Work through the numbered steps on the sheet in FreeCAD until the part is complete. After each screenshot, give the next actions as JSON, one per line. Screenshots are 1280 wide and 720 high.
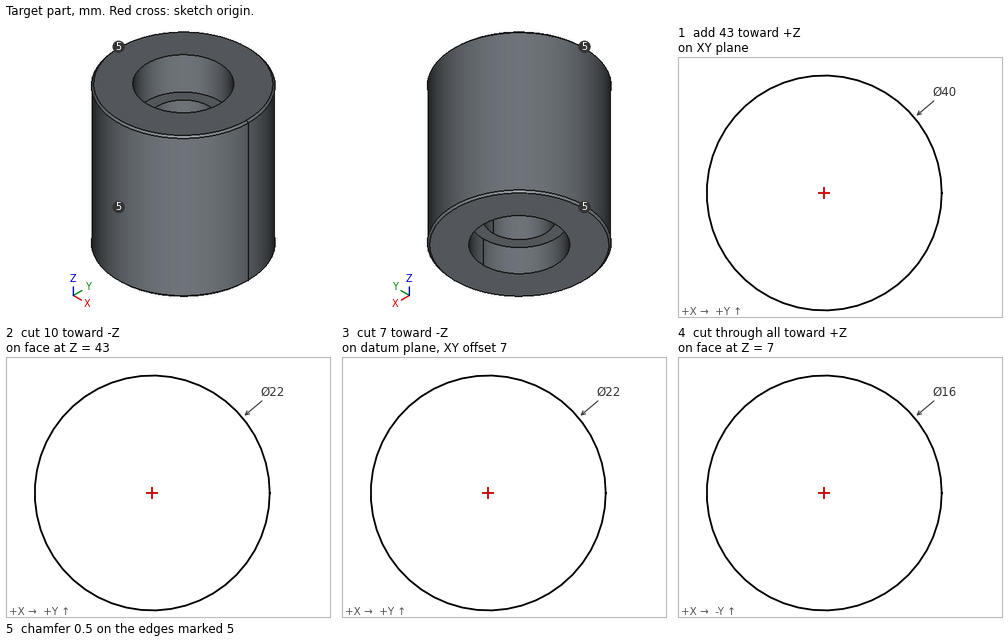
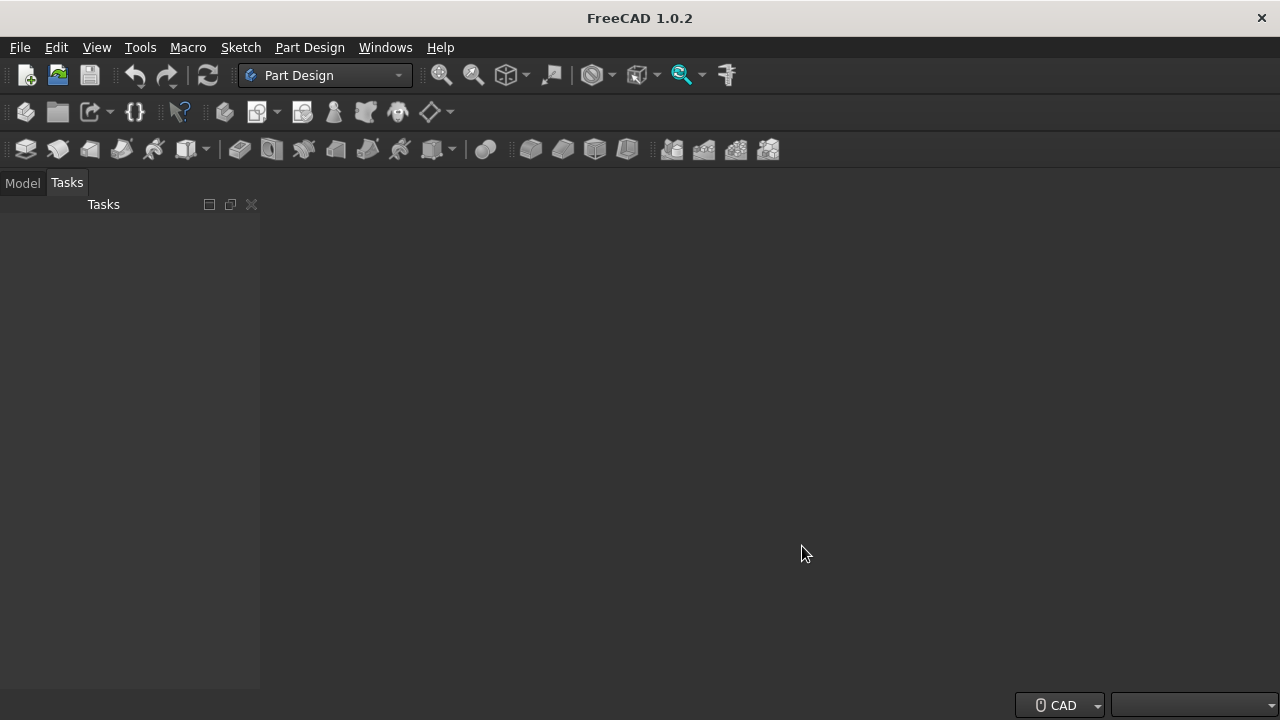
{"action": "left_click", "coordinate": [26, 76]}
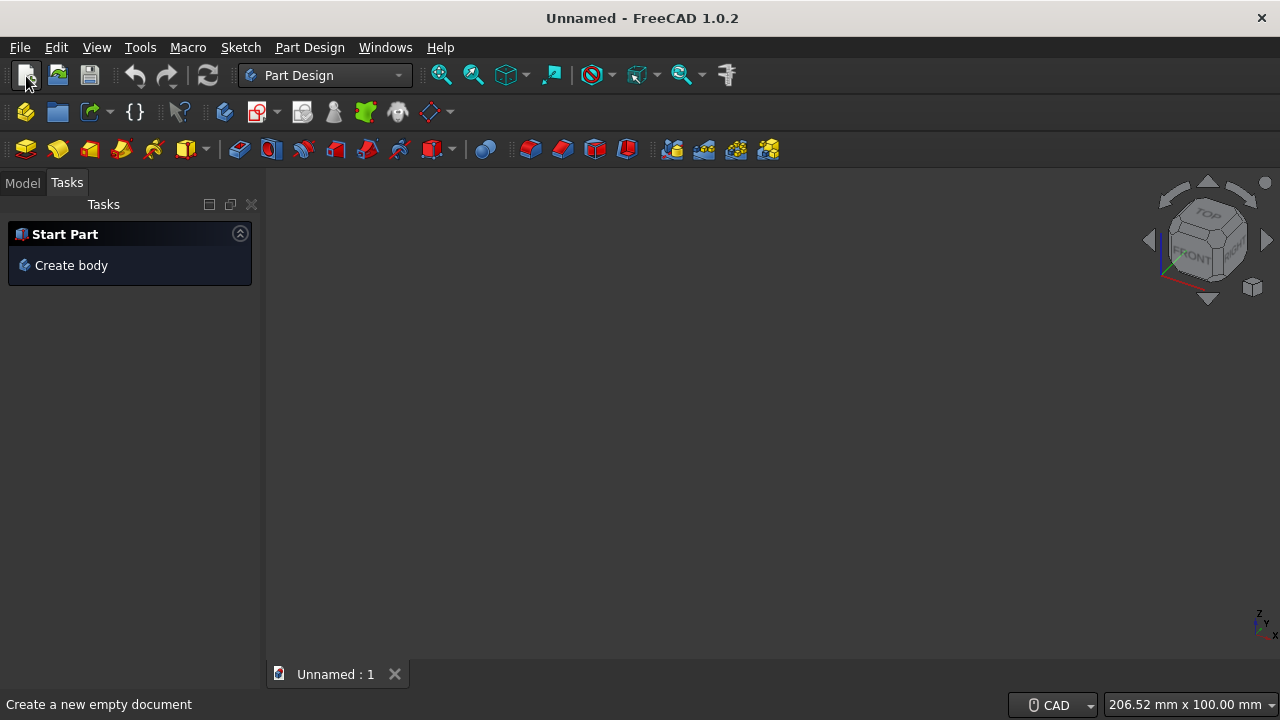
{"action": "left_click", "coordinate": [258, 112]}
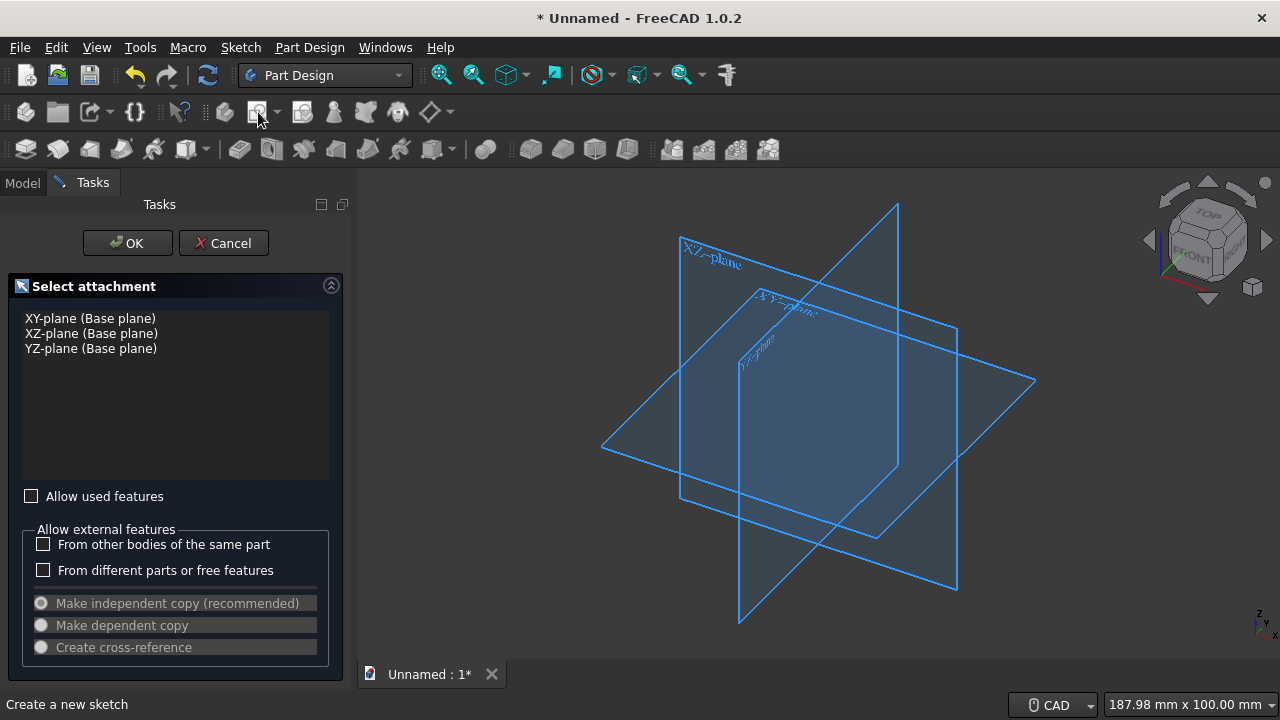
{"action": "left_click", "coordinate": [82, 318]}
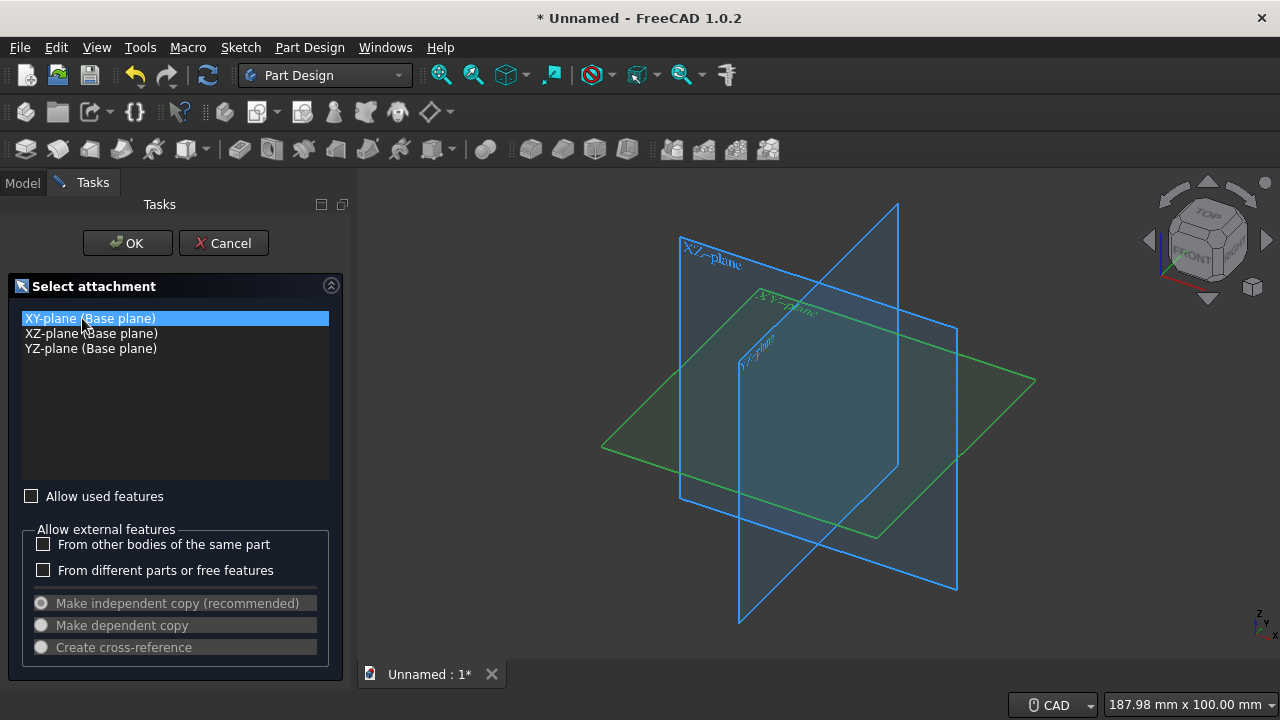
{"action": "left_click", "coordinate": [128, 243]}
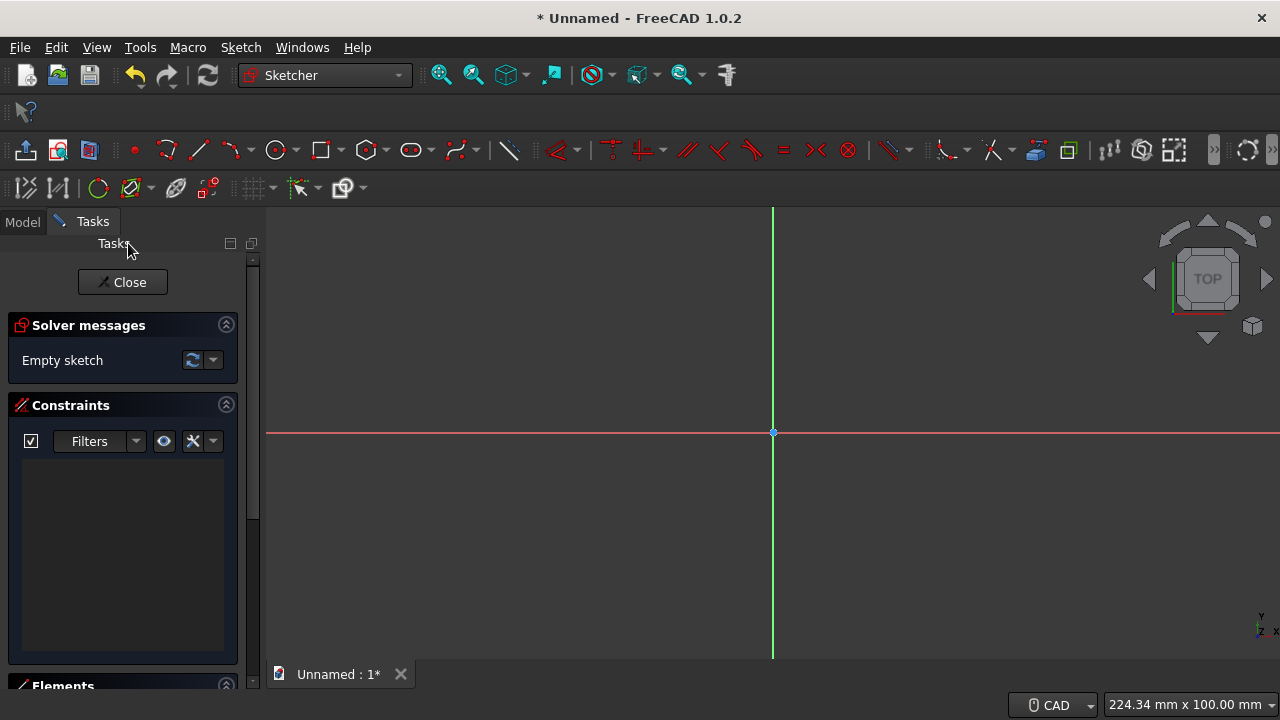
{"action": "scroll", "coordinate": [912, 433], "scroll_direction": "up", "scroll_amount": 2}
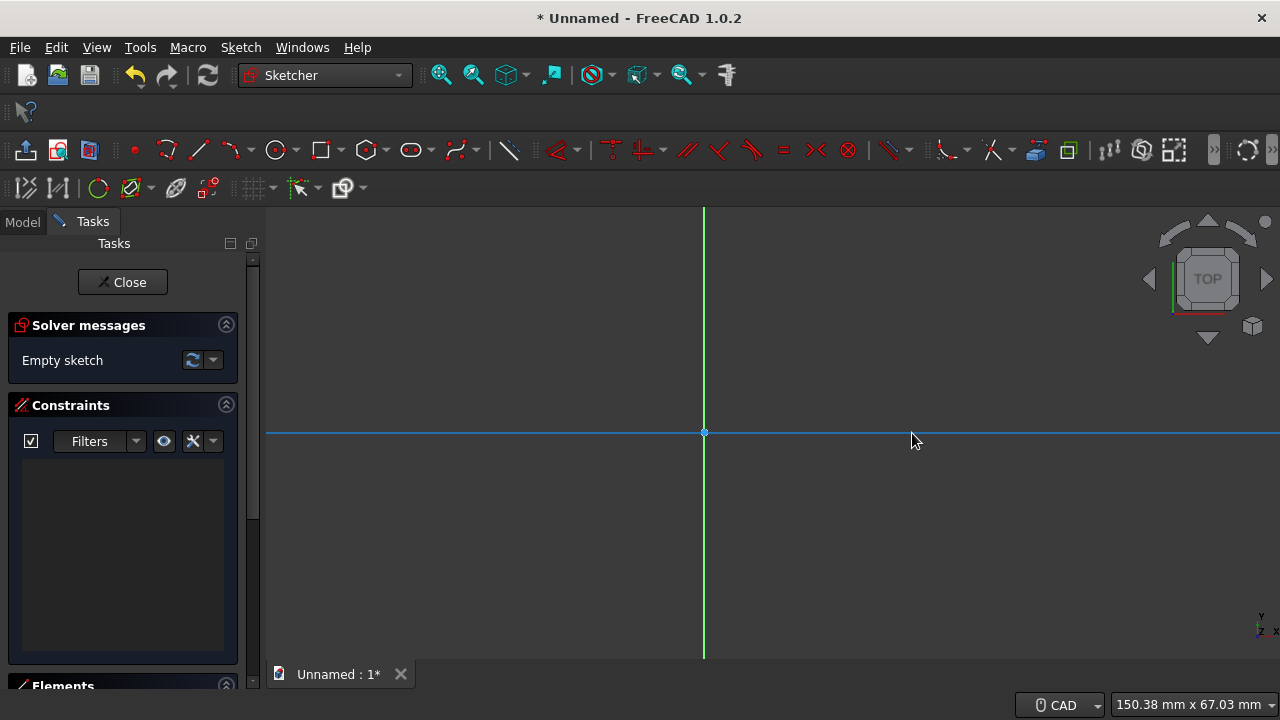
{"action": "left_click", "coordinate": [276, 150]}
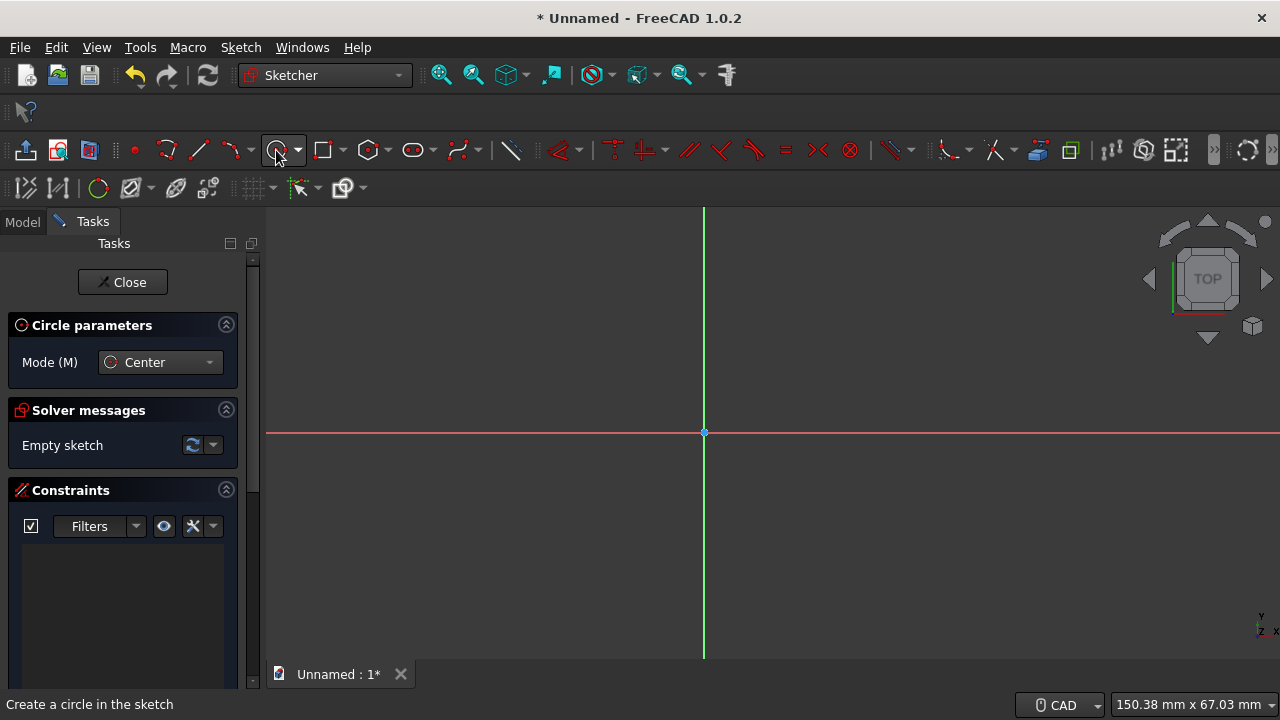
{"action": "left_click", "coordinate": [704, 433]}
{"action": "mouse_move", "coordinate": [800, 337]}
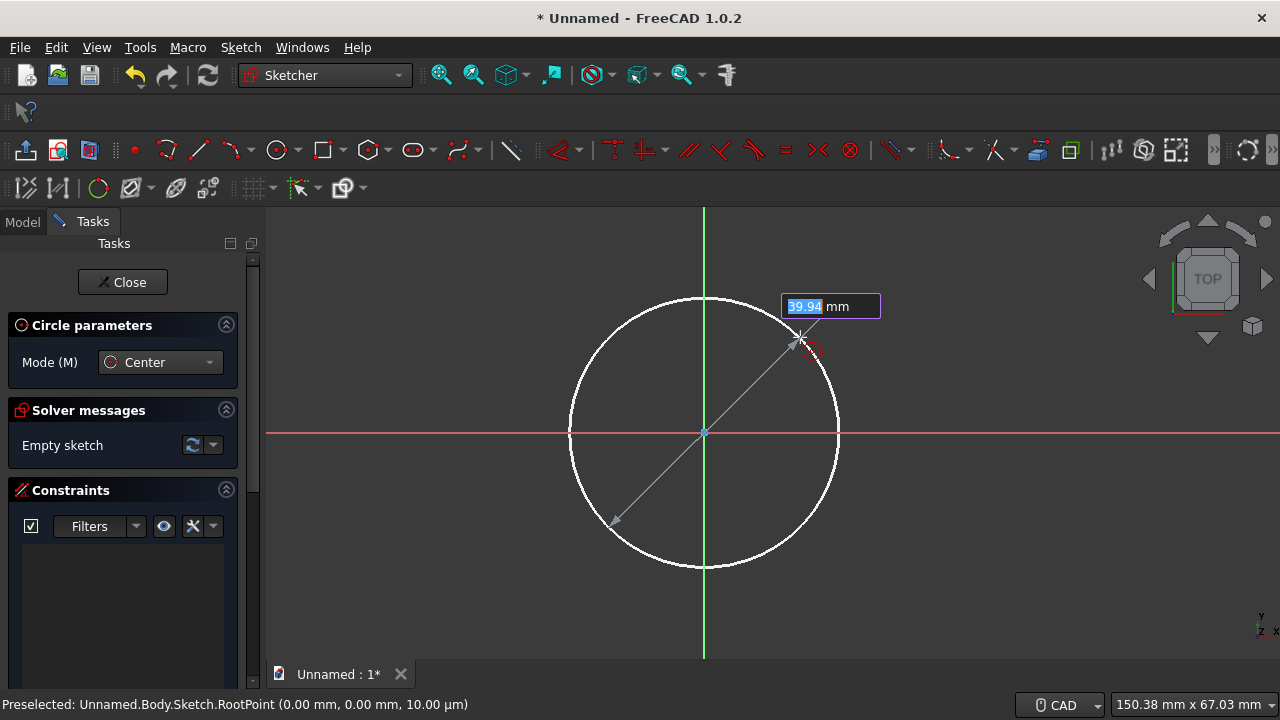
{"action": "type", "text": "40"}
{"action": "key", "text": "Return"}
{"action": "key", "text": "Escape"}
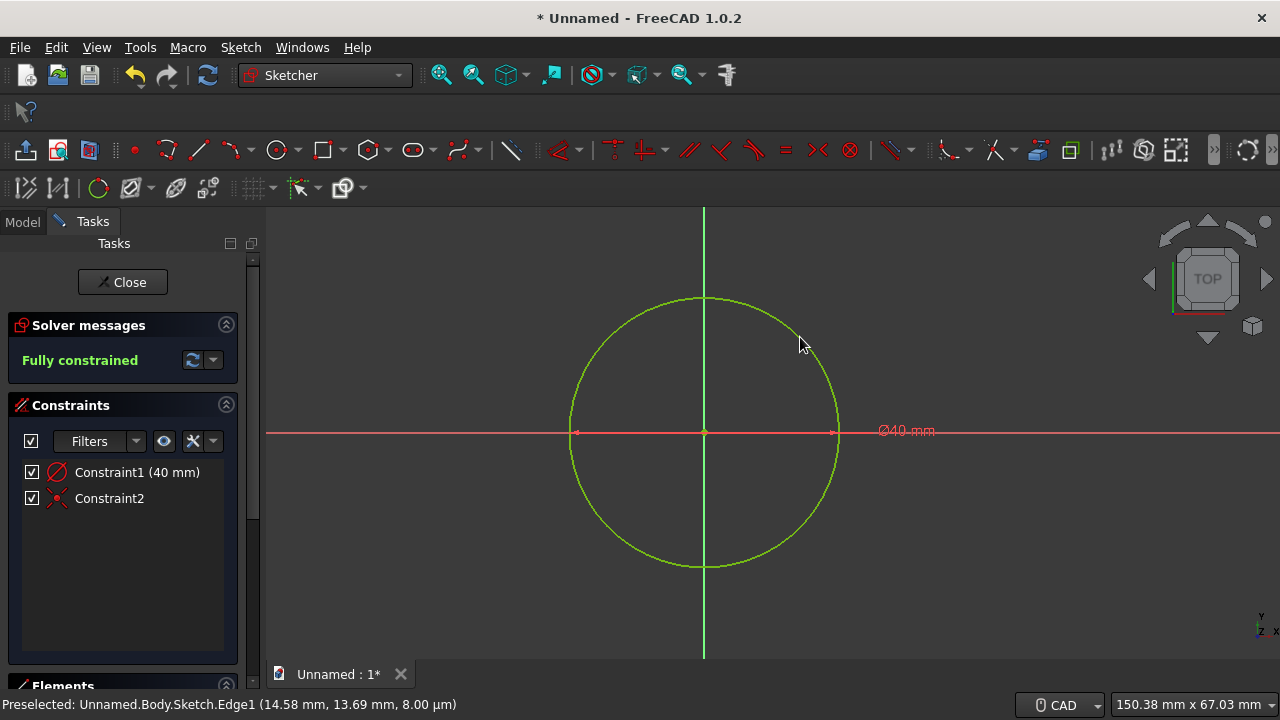
{"action": "left_click", "coordinate": [123, 282]}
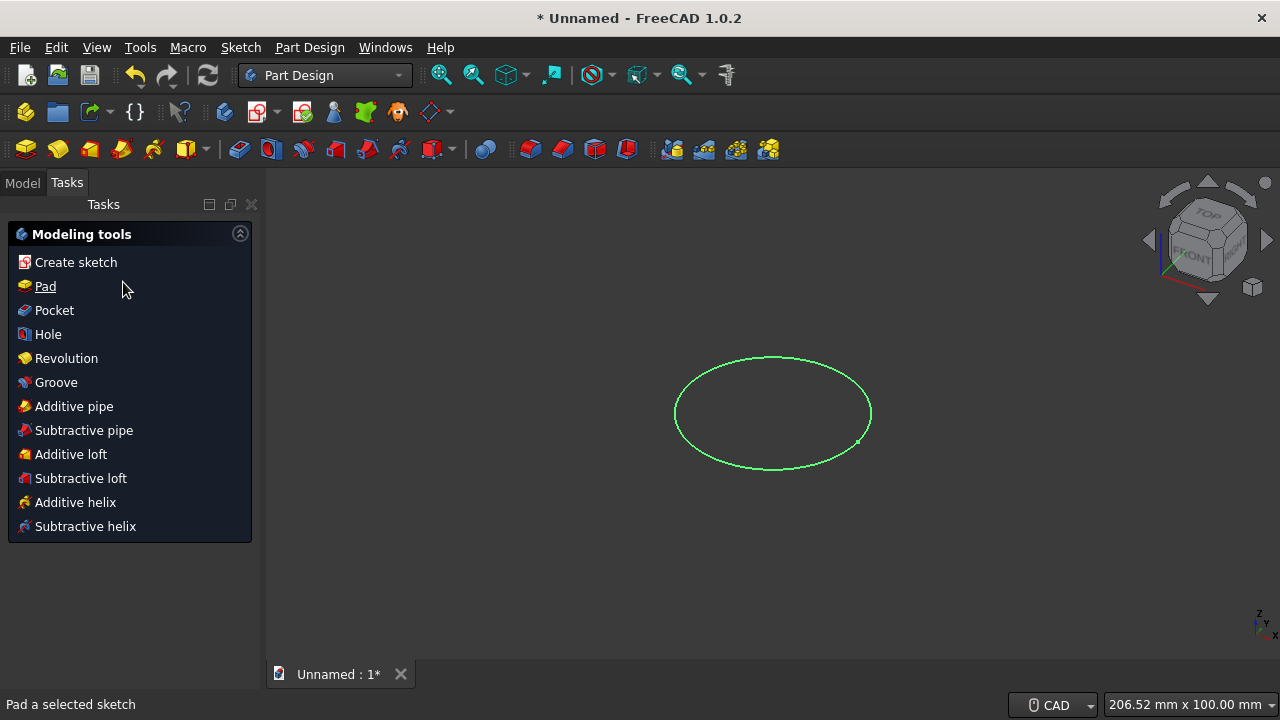
{"action": "left_click", "coordinate": [26, 150]}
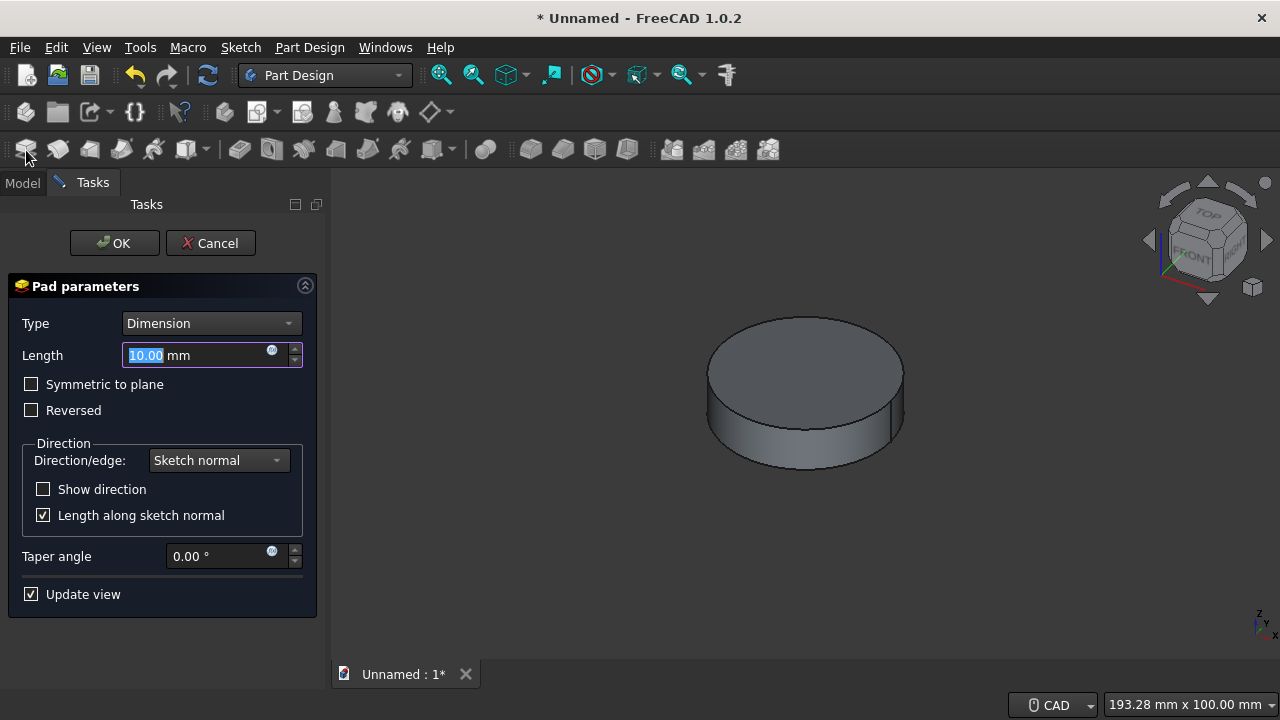
{"action": "type", "text": "43"}
{"action": "key", "text": "Tab"}